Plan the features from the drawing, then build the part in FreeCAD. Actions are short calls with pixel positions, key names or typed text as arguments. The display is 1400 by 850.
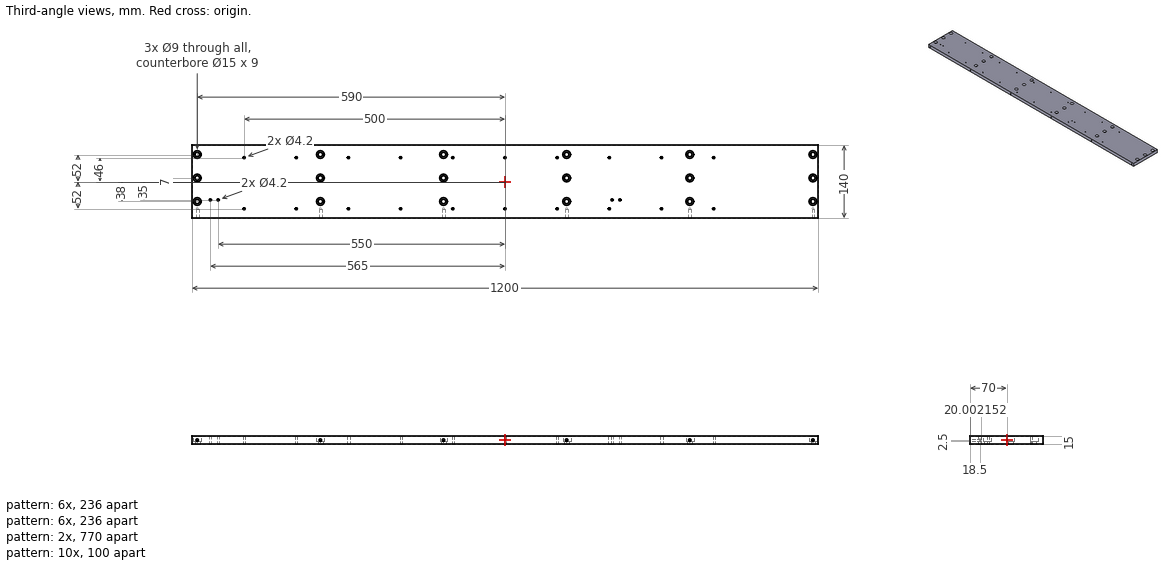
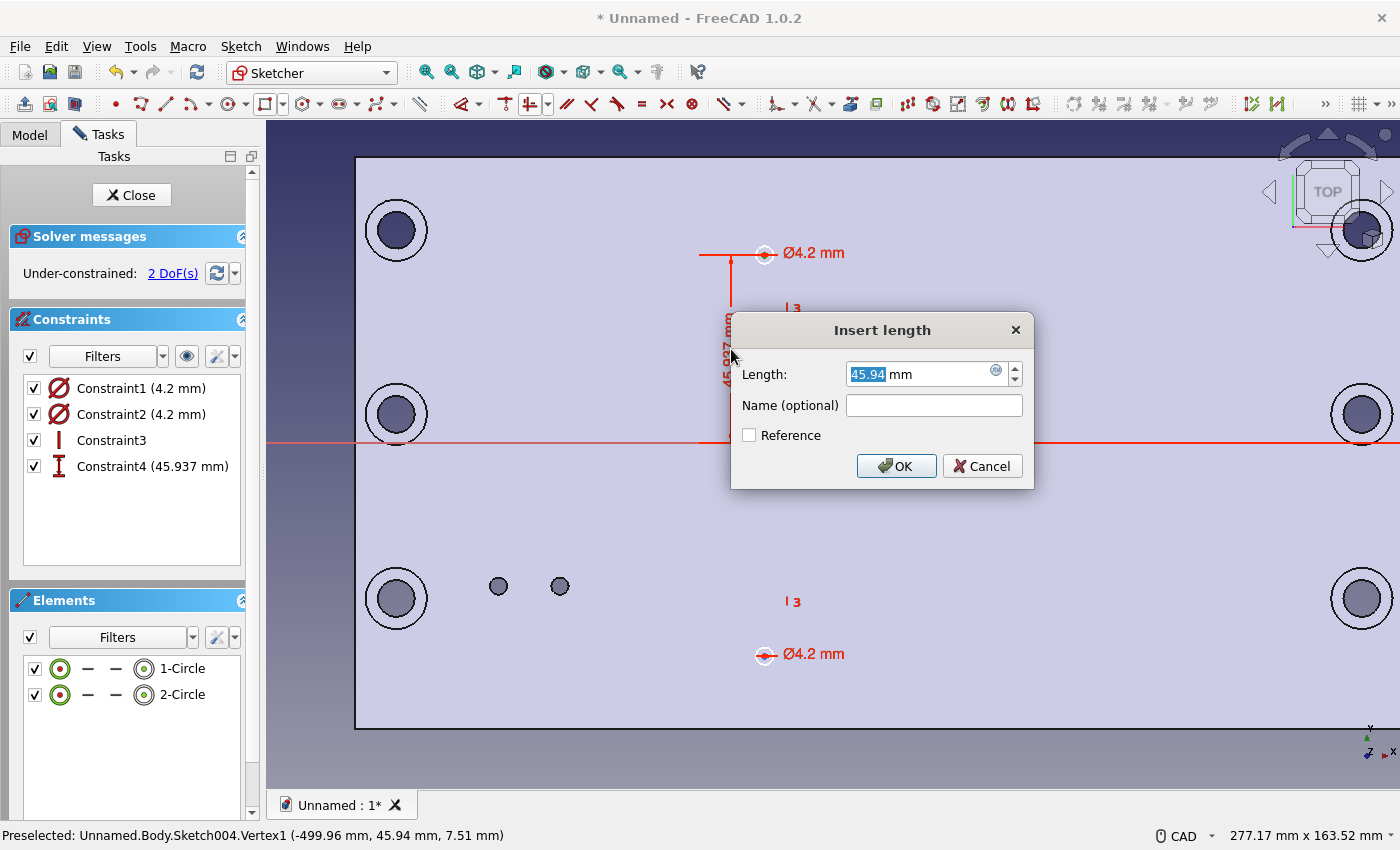
text(46)
key(Return)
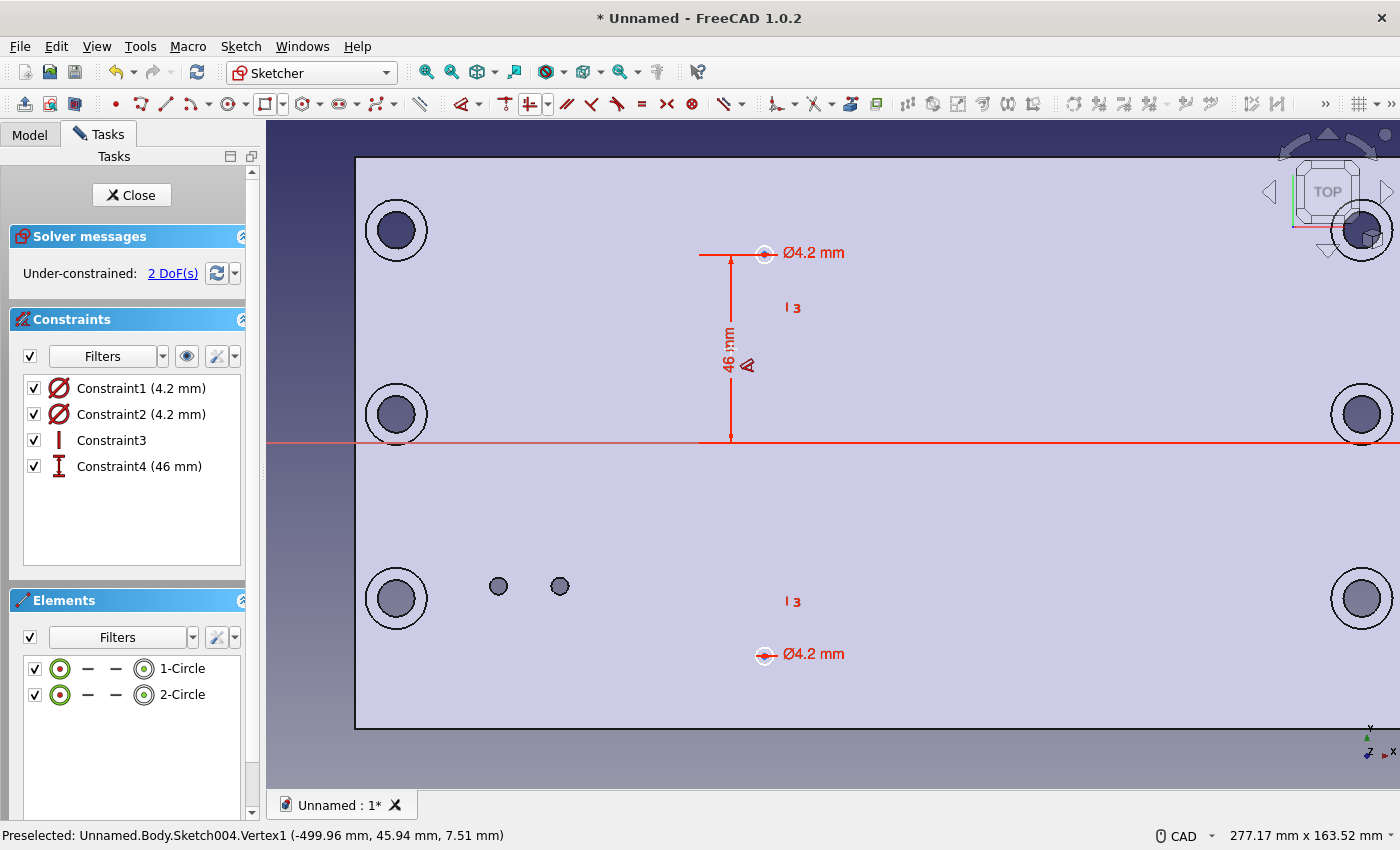
click(765, 656)
click(731, 550)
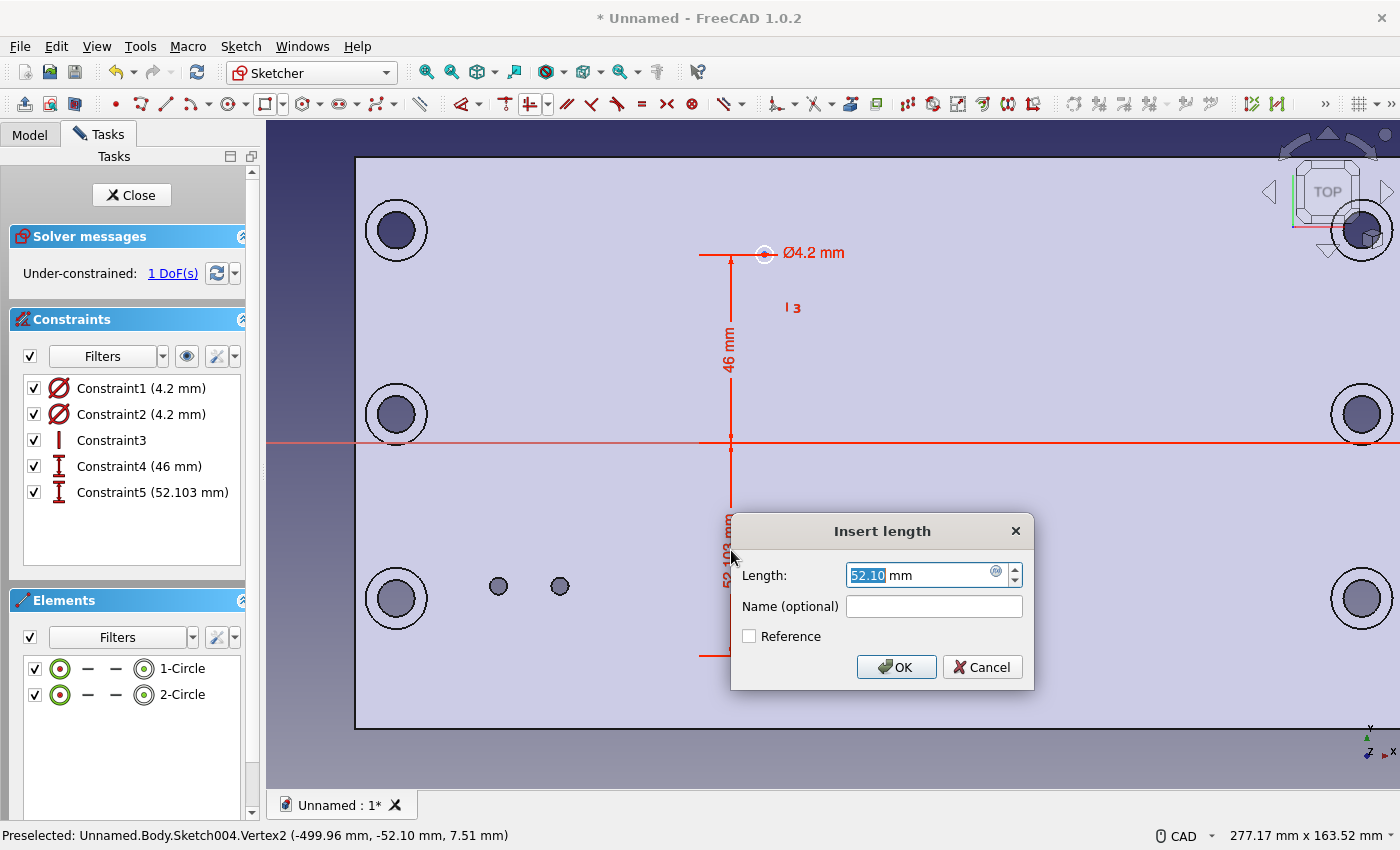
text(52)
key(Return)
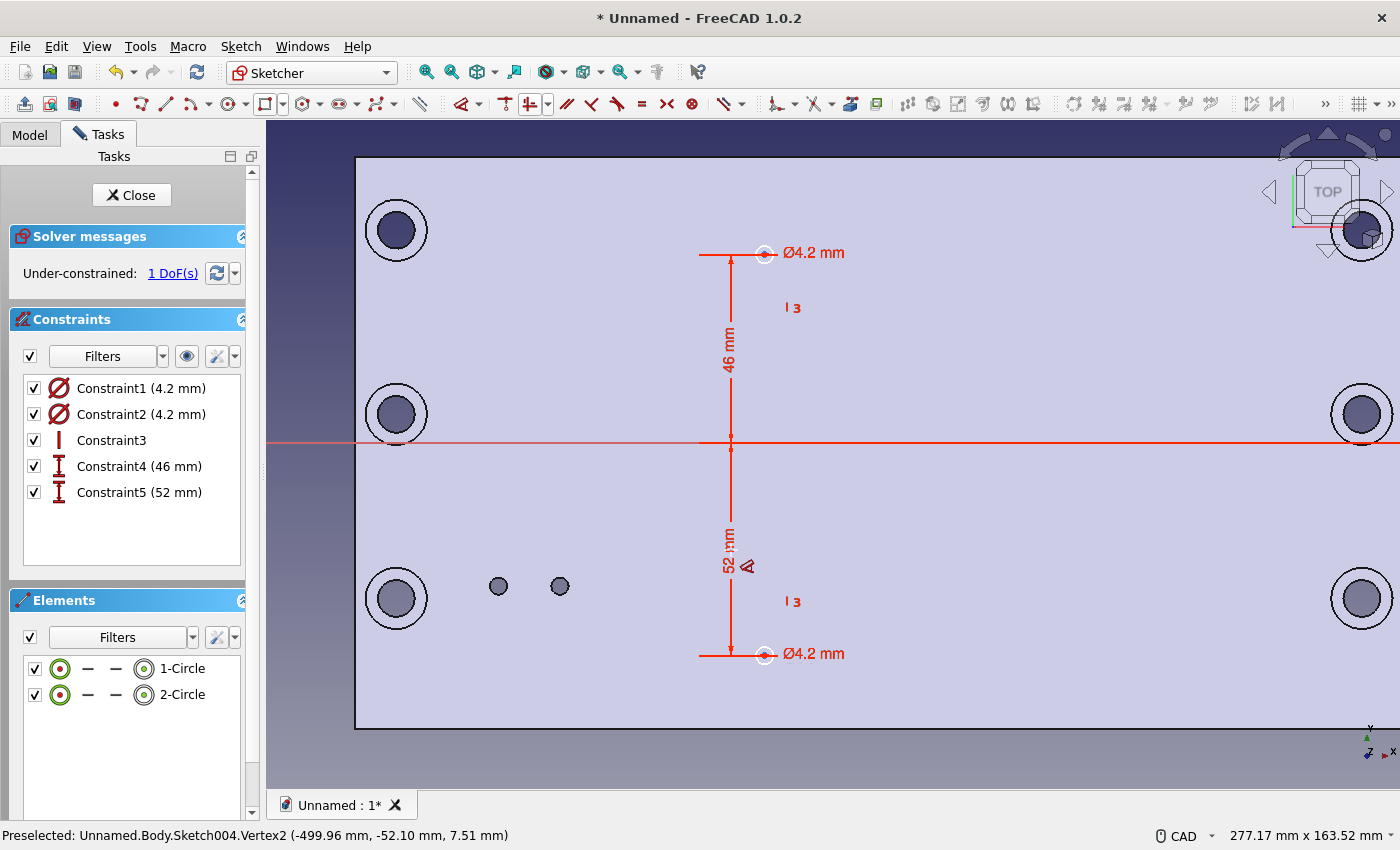
click(765, 255)
click(1000, 221)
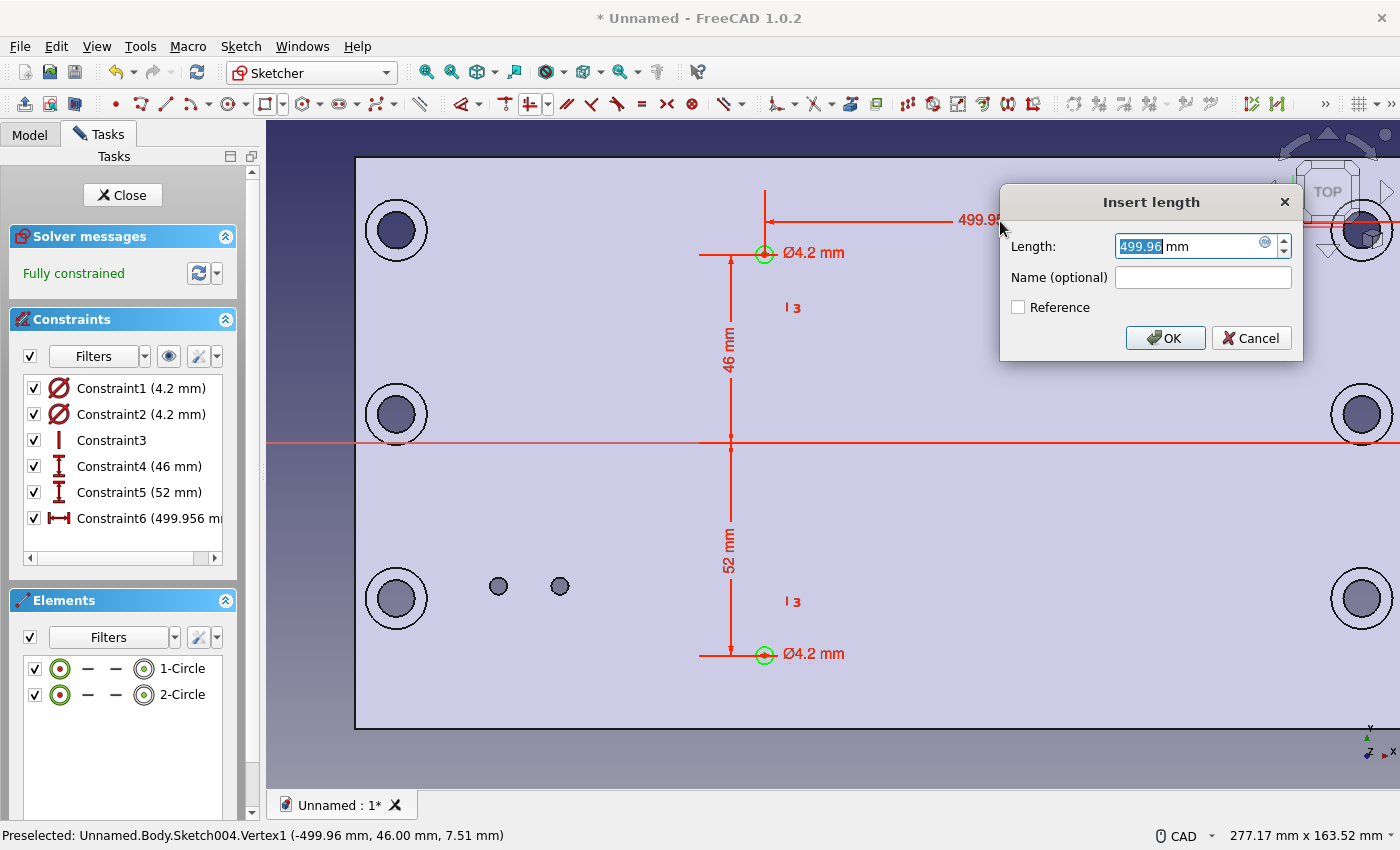
text(500)
key(Return)
key(Escape)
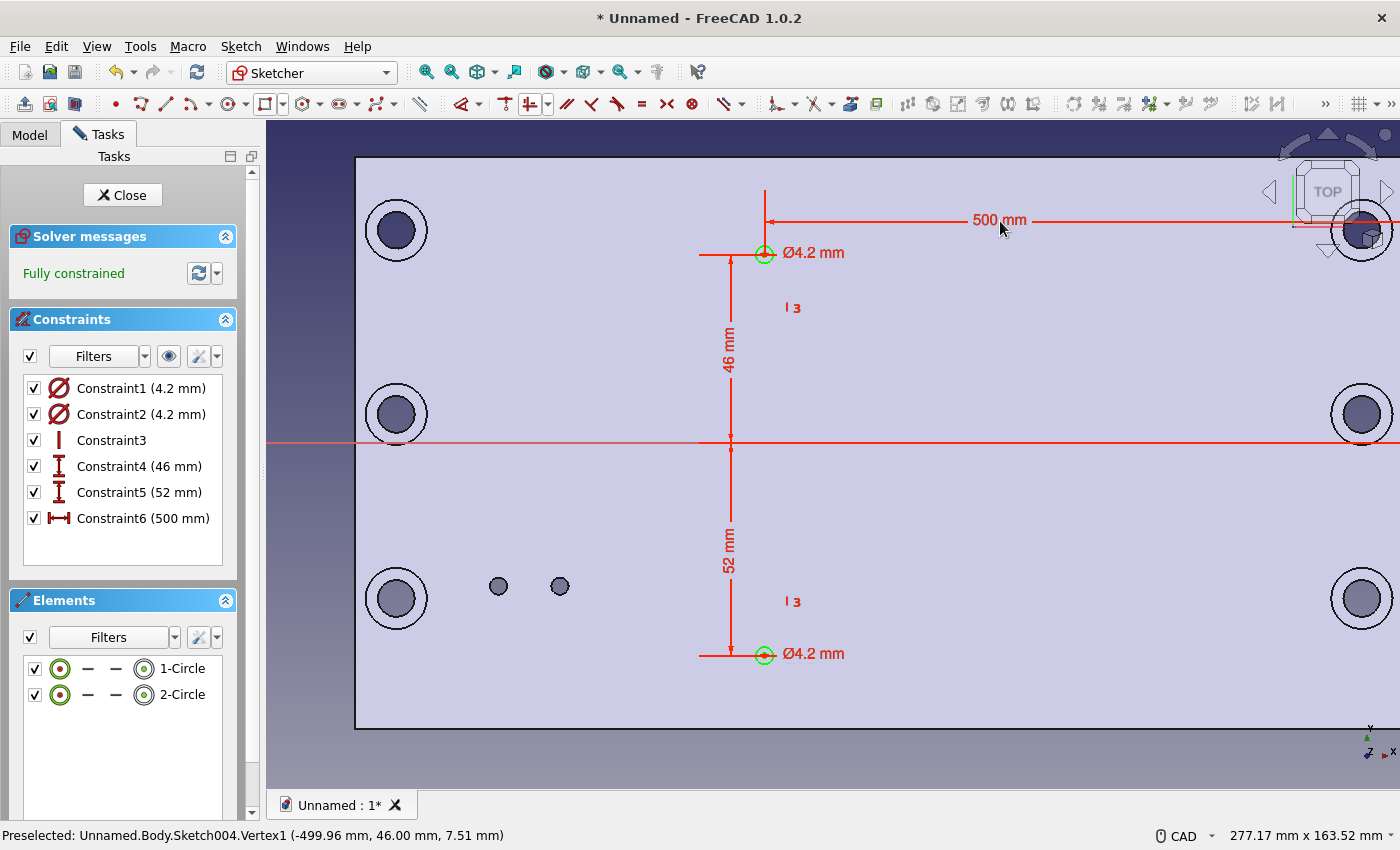
click(123, 195)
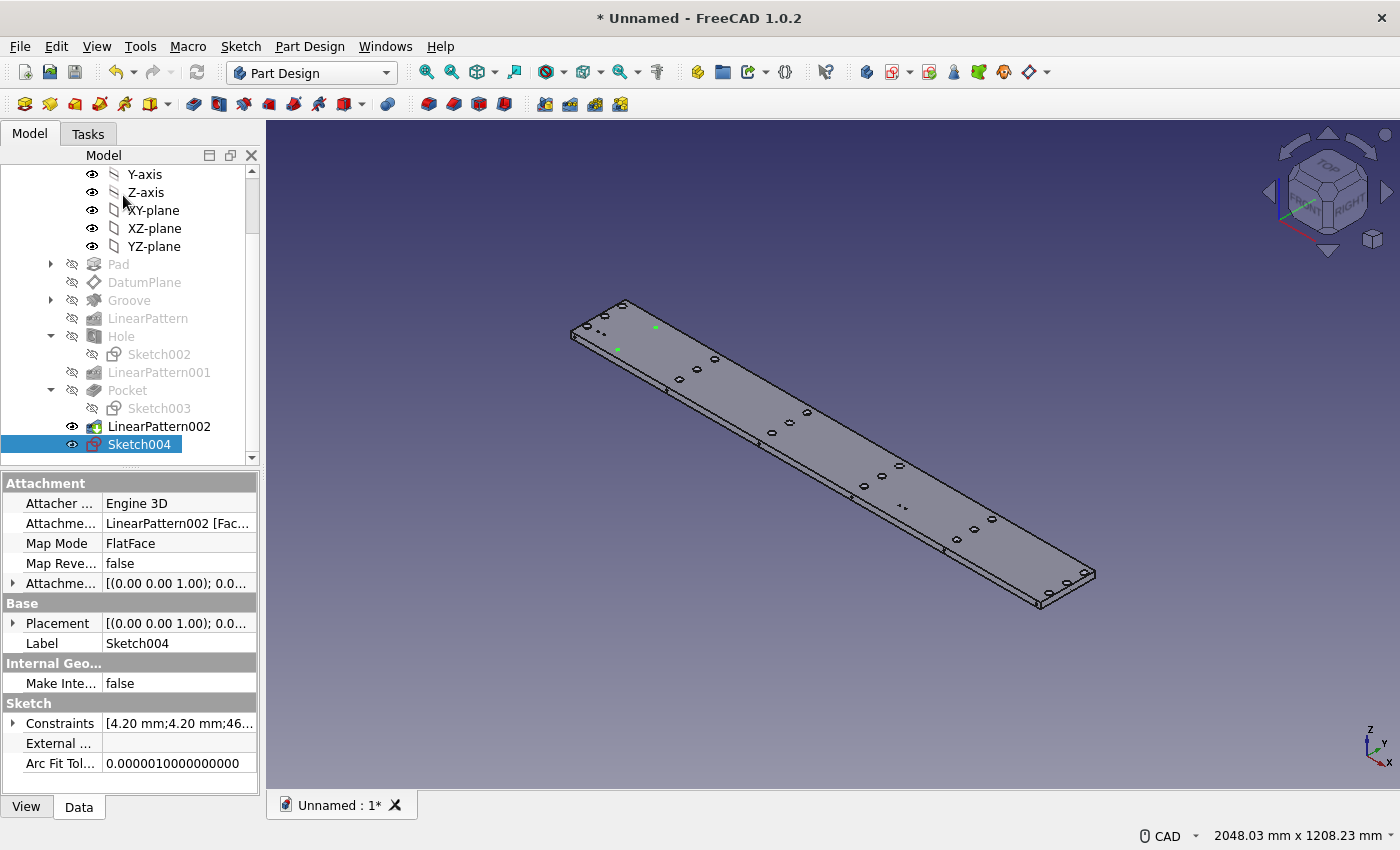
click(194, 104)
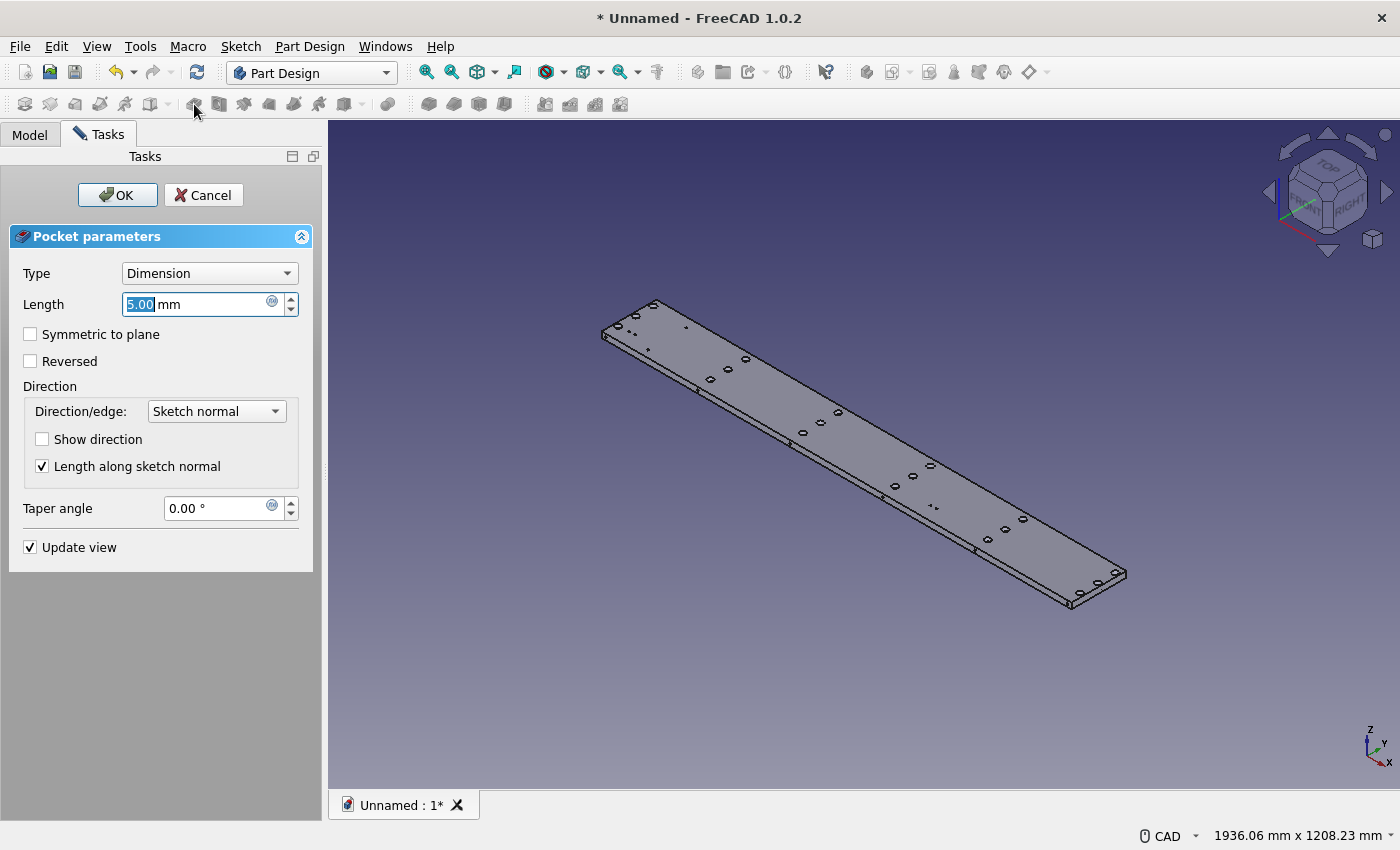
click(210, 274)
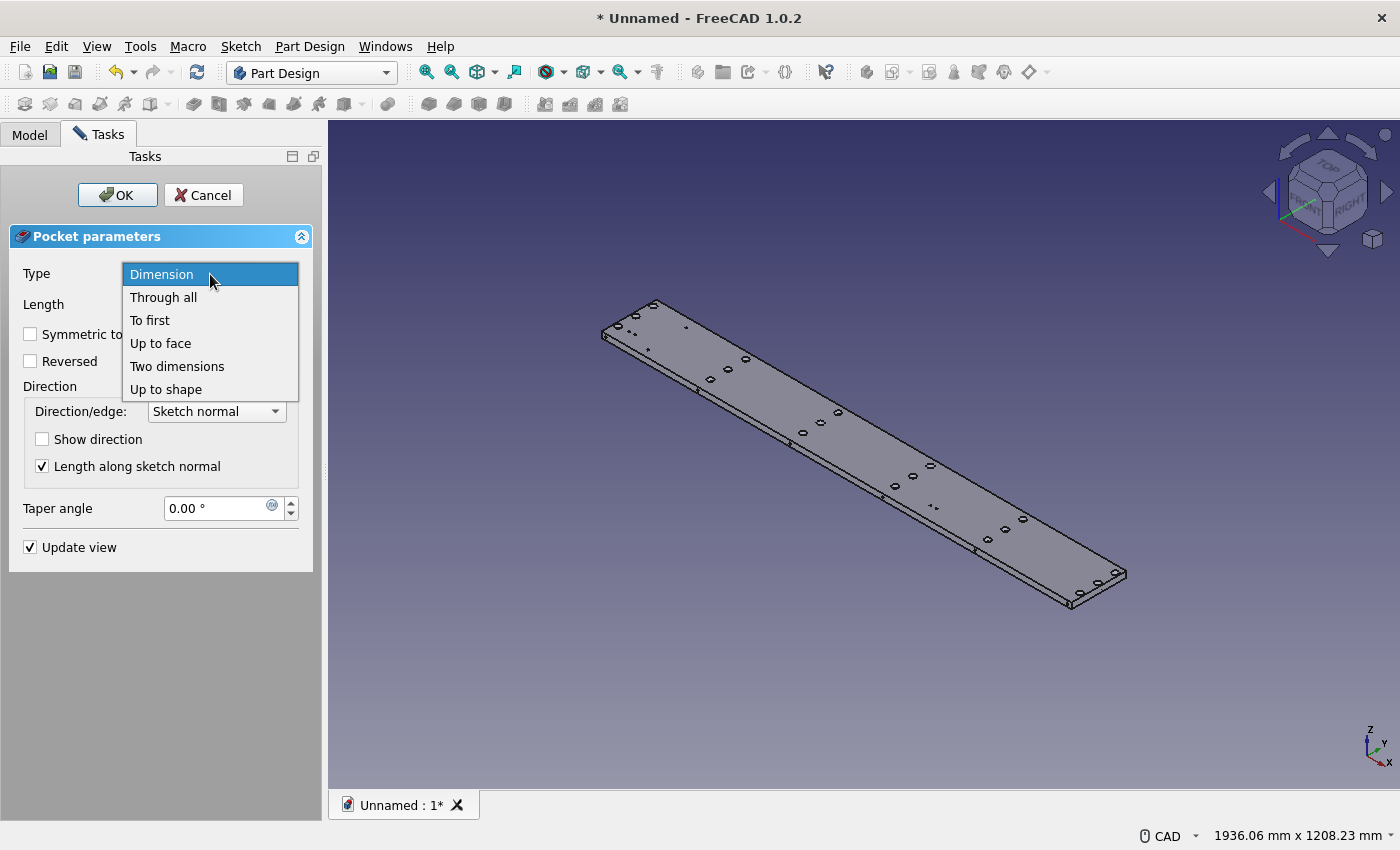
click(208, 298)